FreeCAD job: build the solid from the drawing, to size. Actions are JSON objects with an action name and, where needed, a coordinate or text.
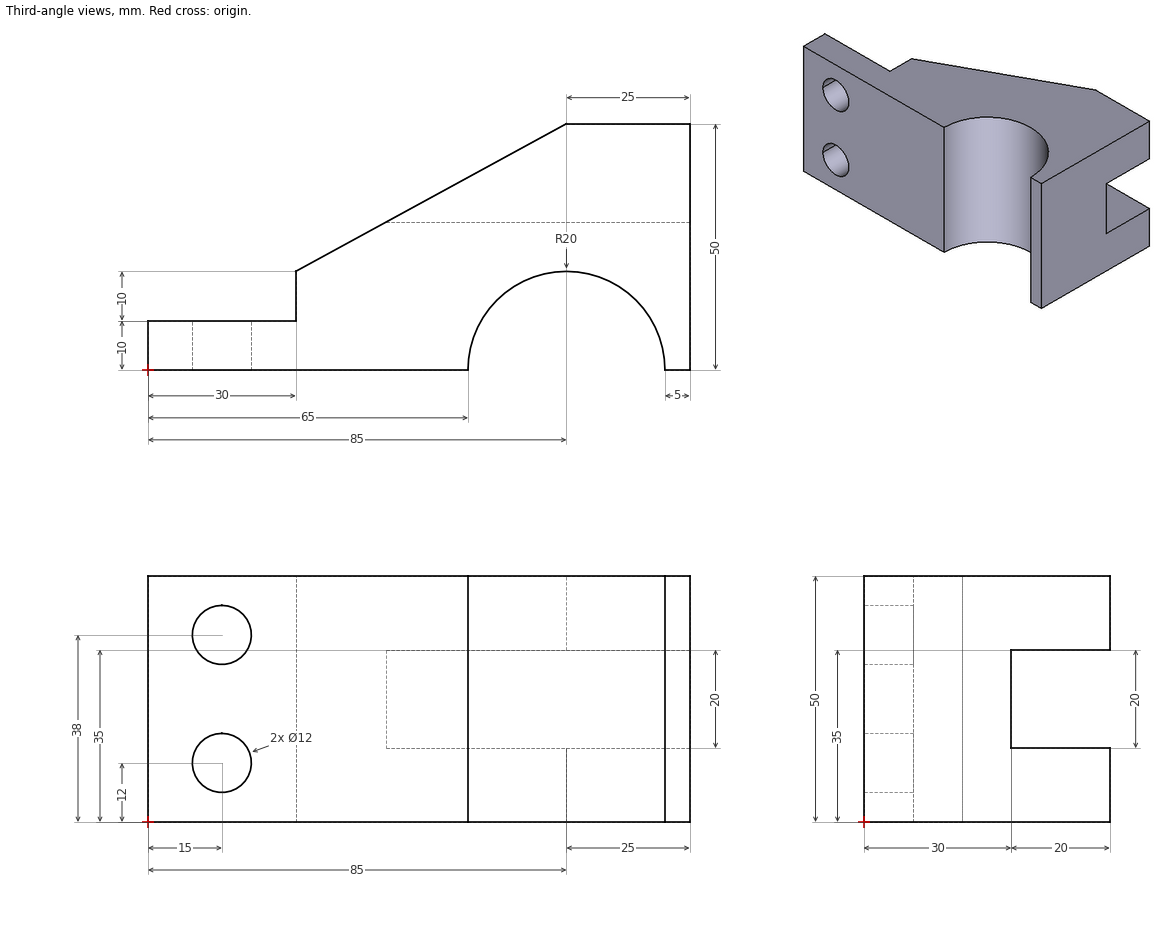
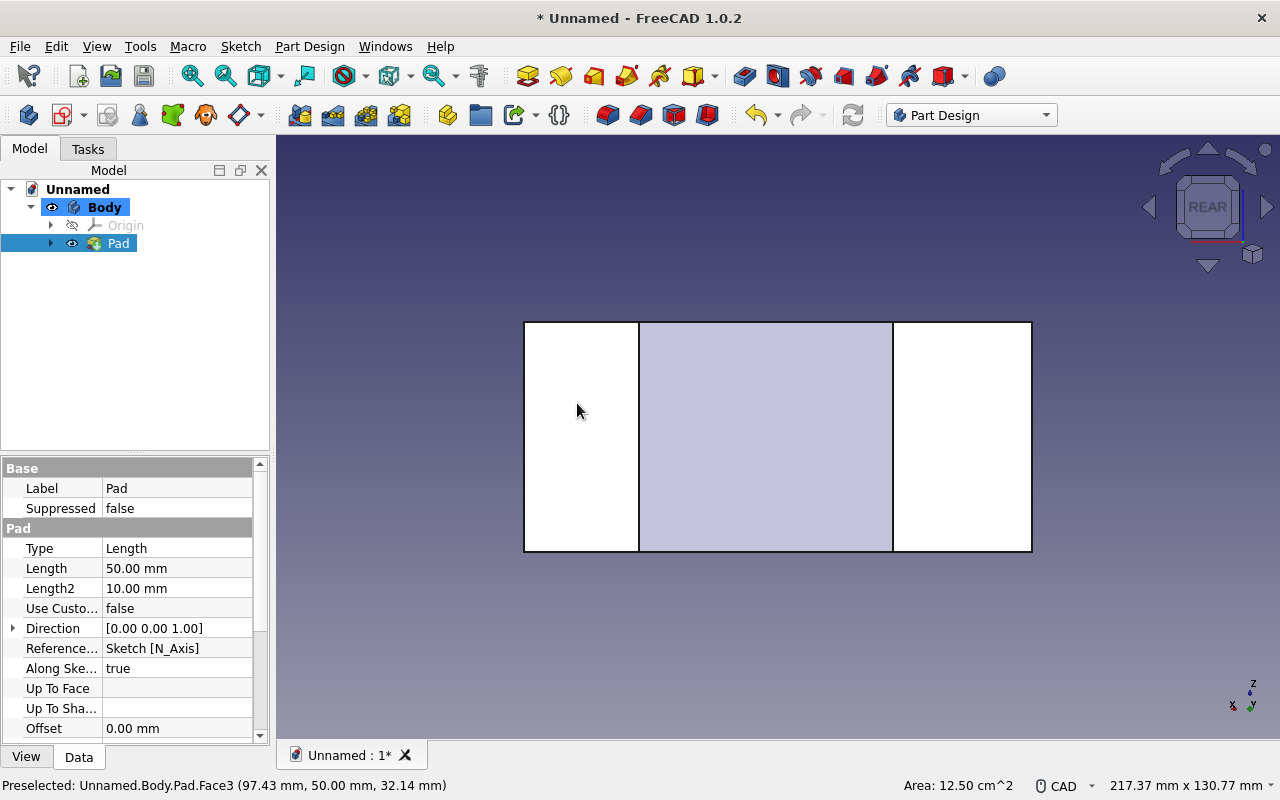
{"action": "left_click", "coordinate": [62, 116]}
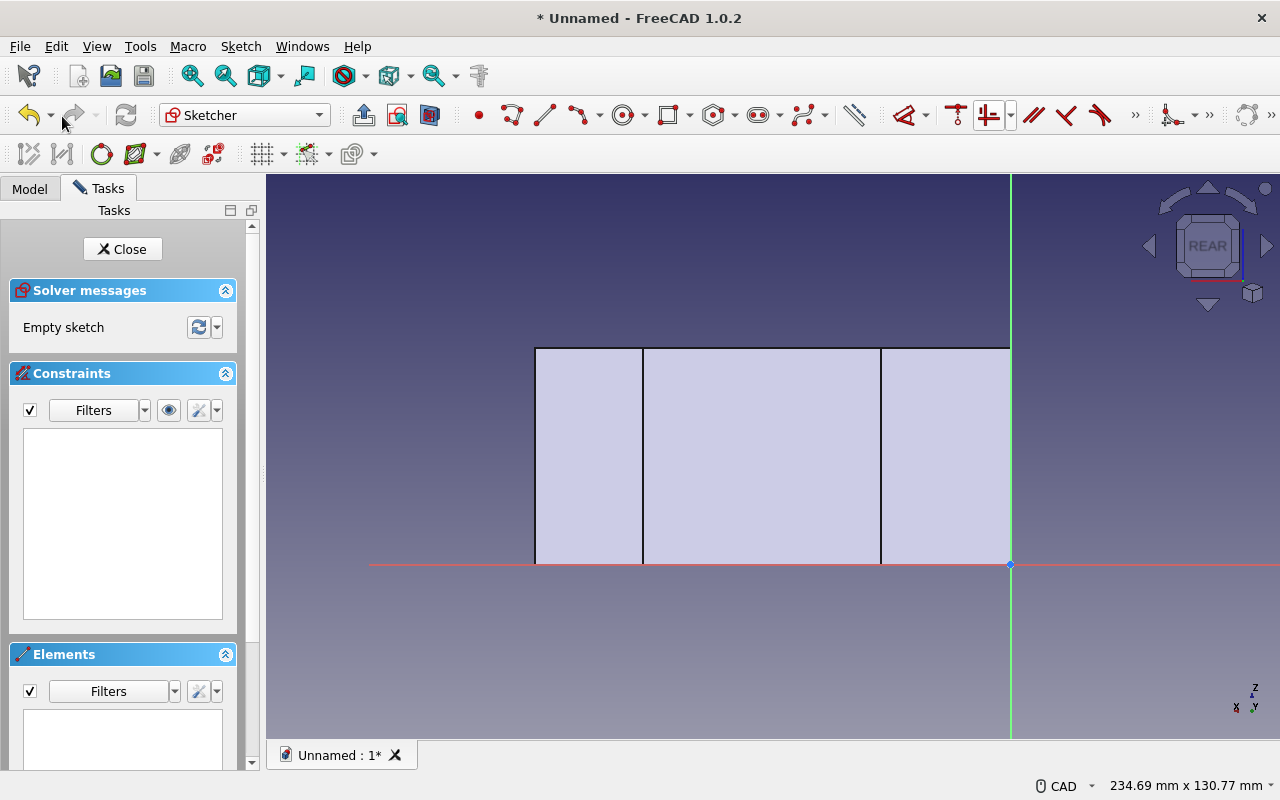
{"action": "scroll", "coordinate": [552, 456], "scroll_direction": "up", "scroll_amount": 7}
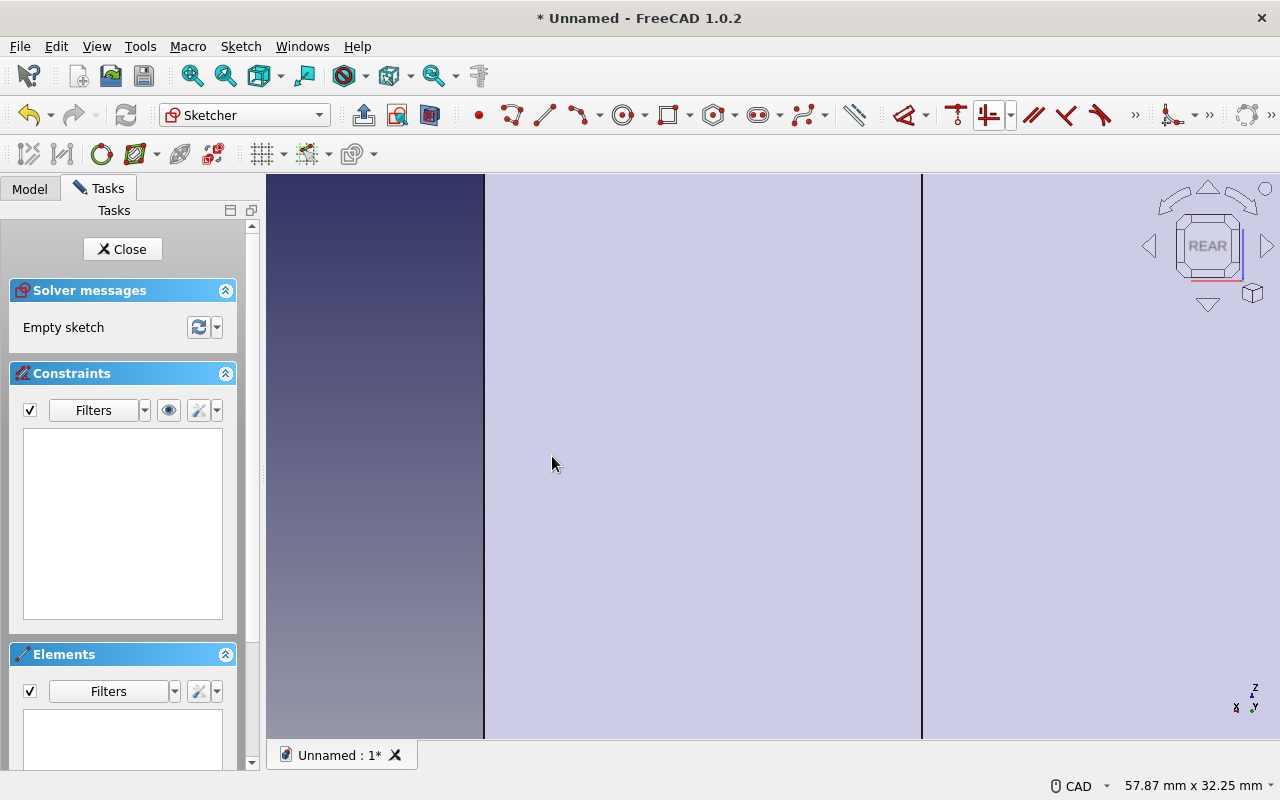
{"action": "left_click", "coordinate": [668, 116]}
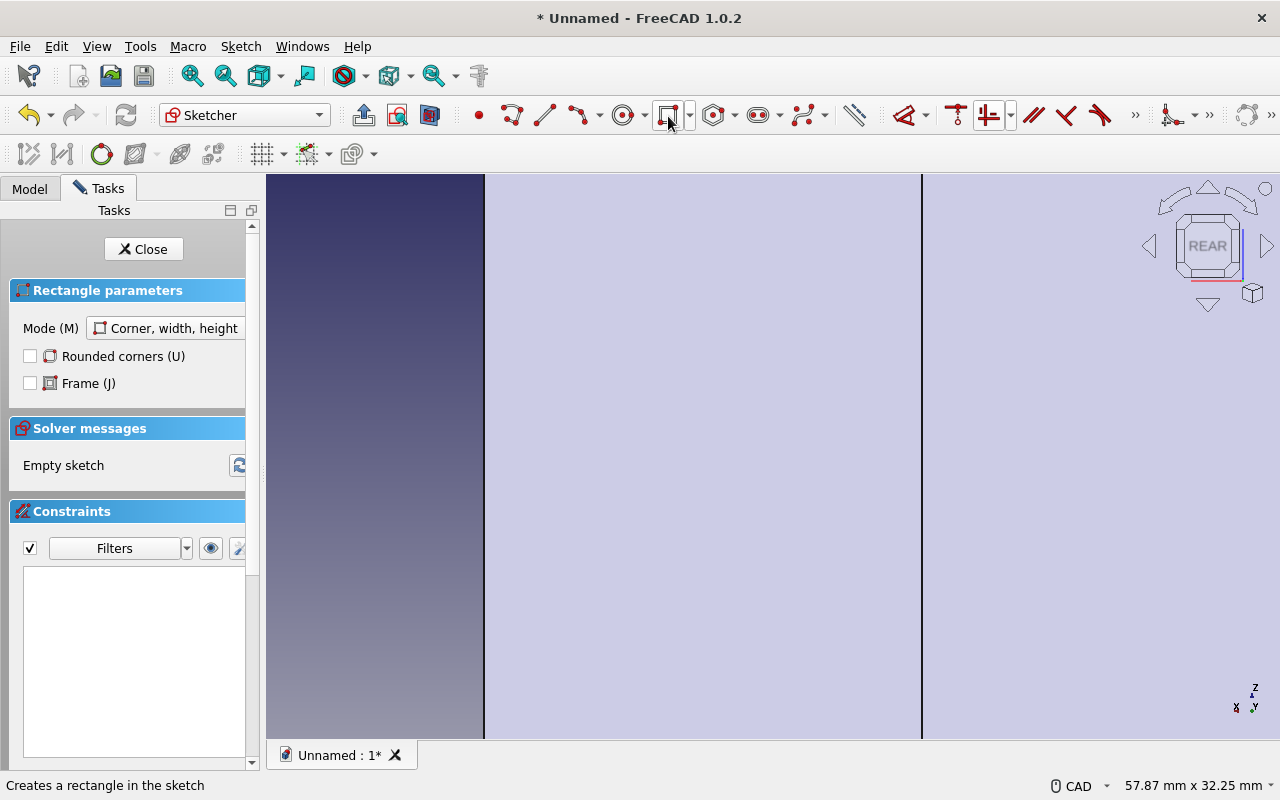
{"action": "left_click", "coordinate": [484, 281]}
{"action": "left_click", "coordinate": [922, 632]}
{"action": "key", "text": "Escape"}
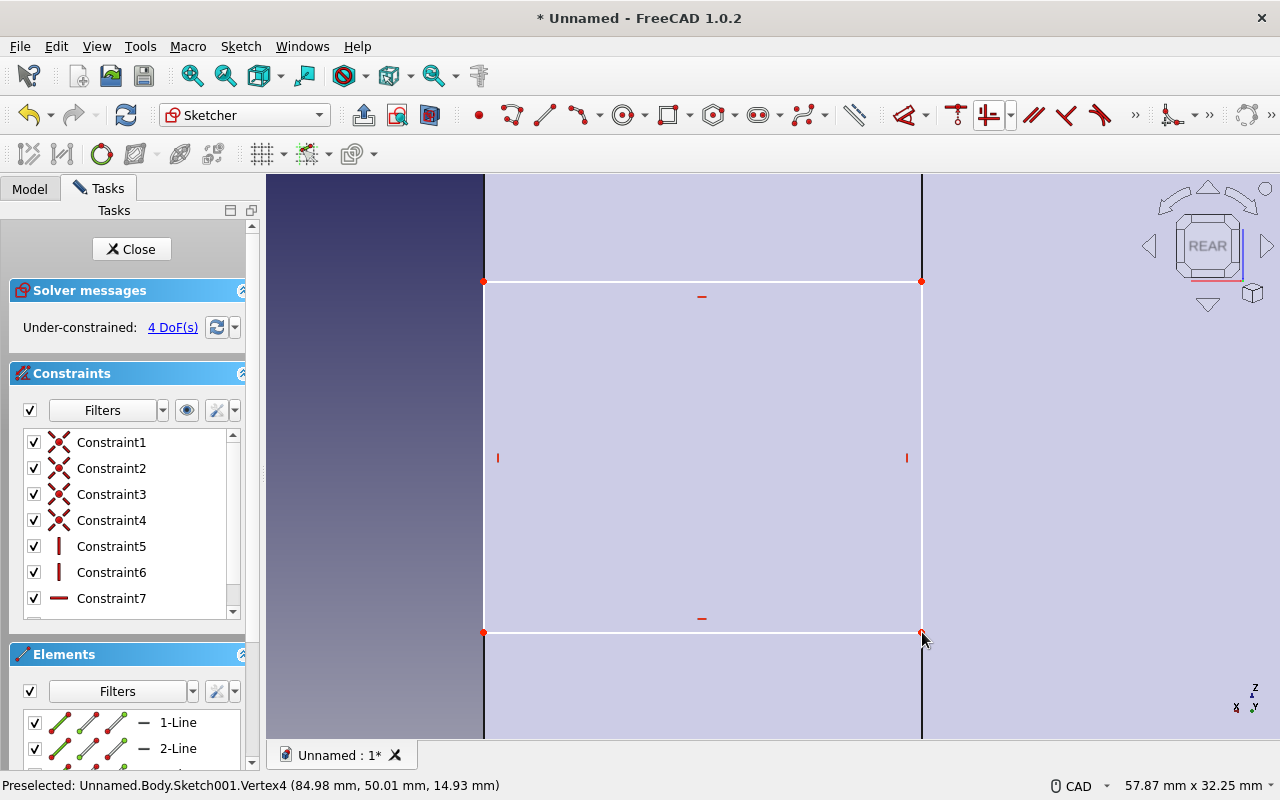
{"action": "left_click", "coordinate": [904, 116]}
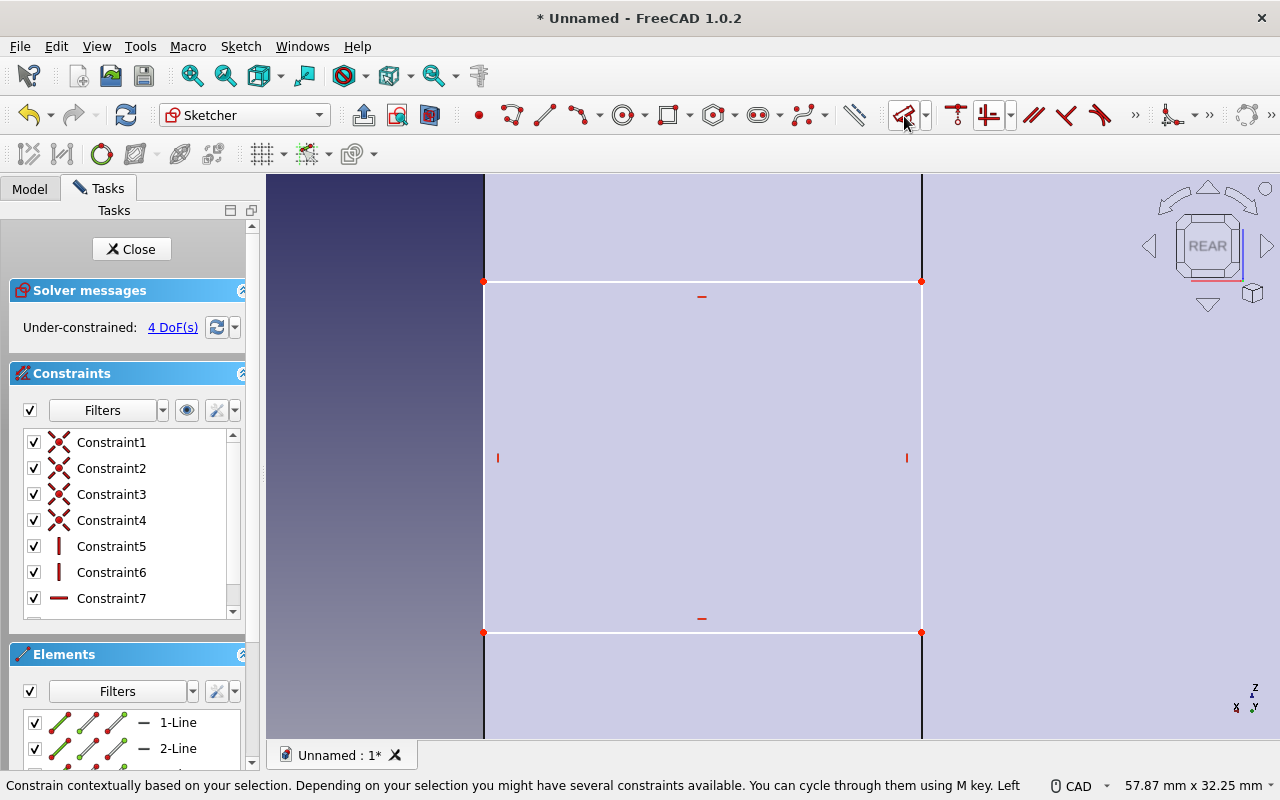
{"action": "left_click", "coordinate": [484, 387]}
{"action": "left_click", "coordinate": [450, 457]}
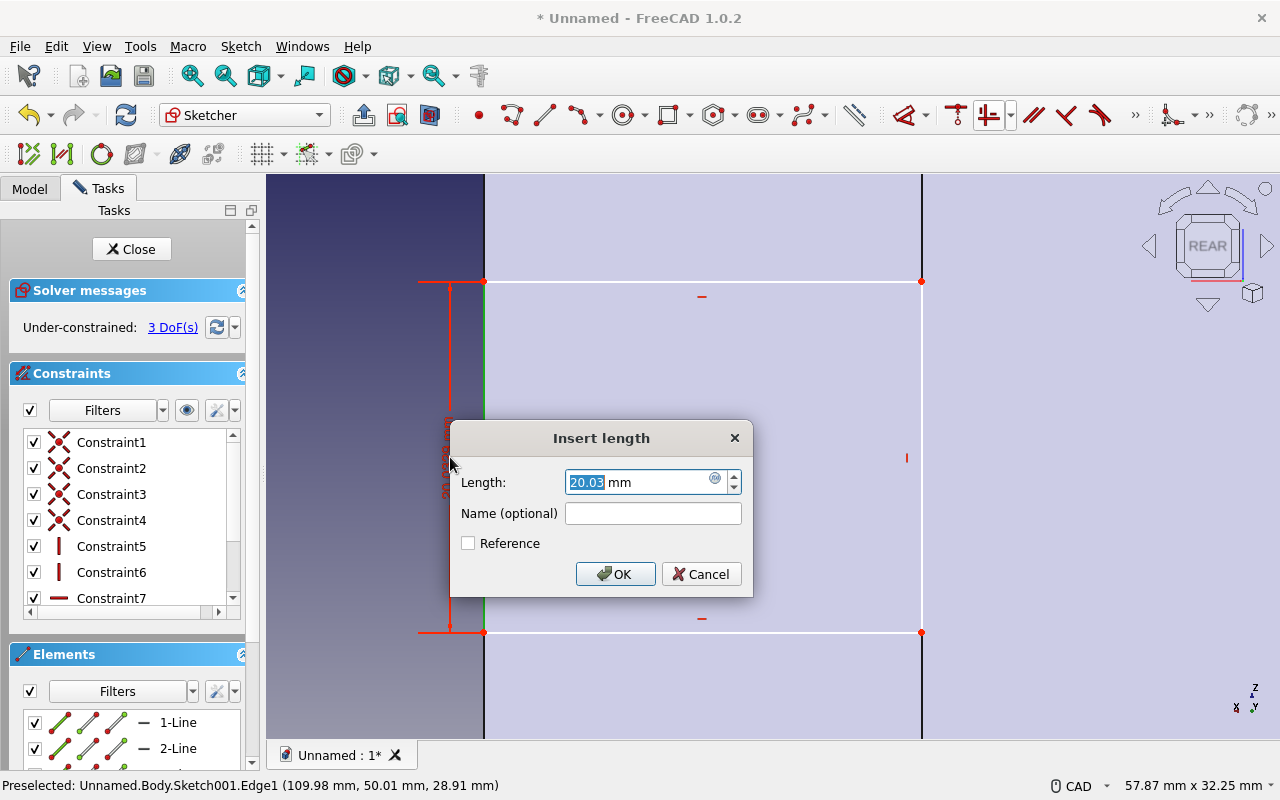
{"action": "type", "text": "20"}
{"action": "key", "text": "Return"}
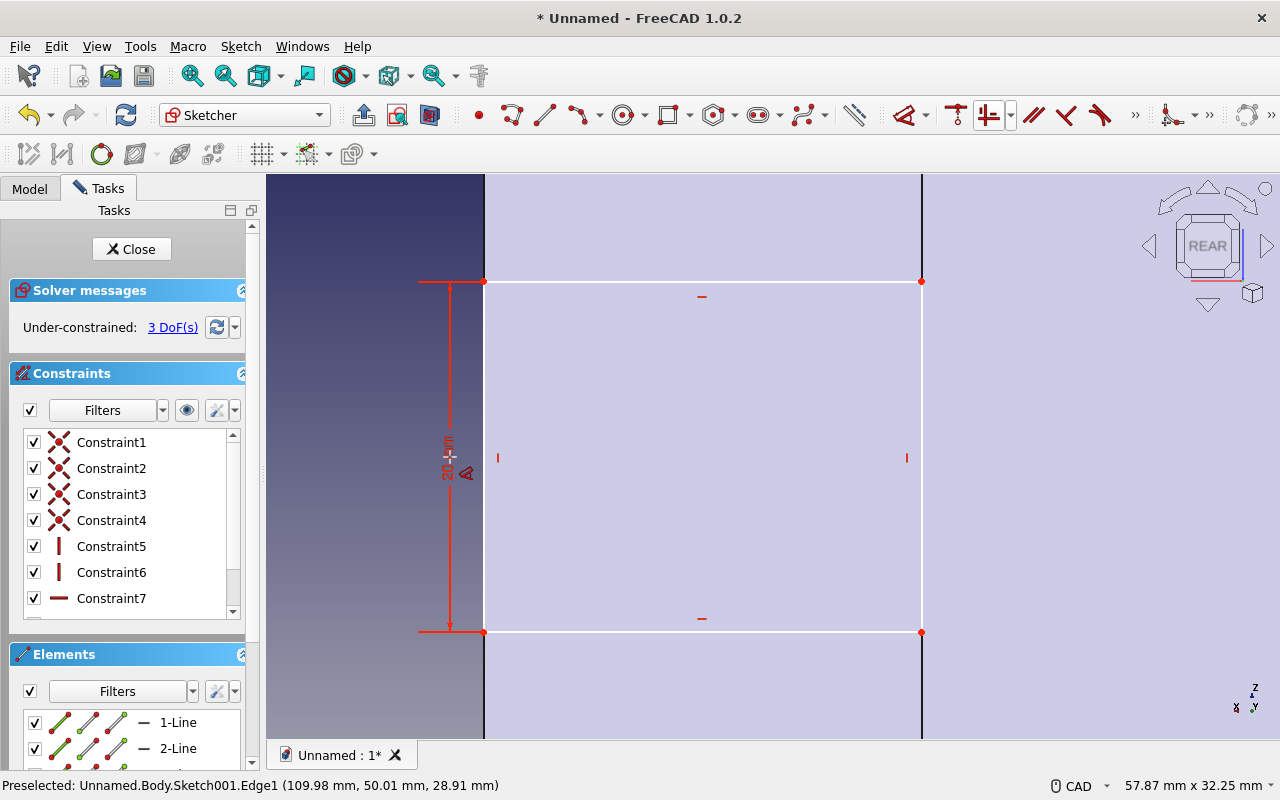
{"action": "left_click", "coordinate": [615, 632]}
{"action": "left_click", "coordinate": [703, 666]}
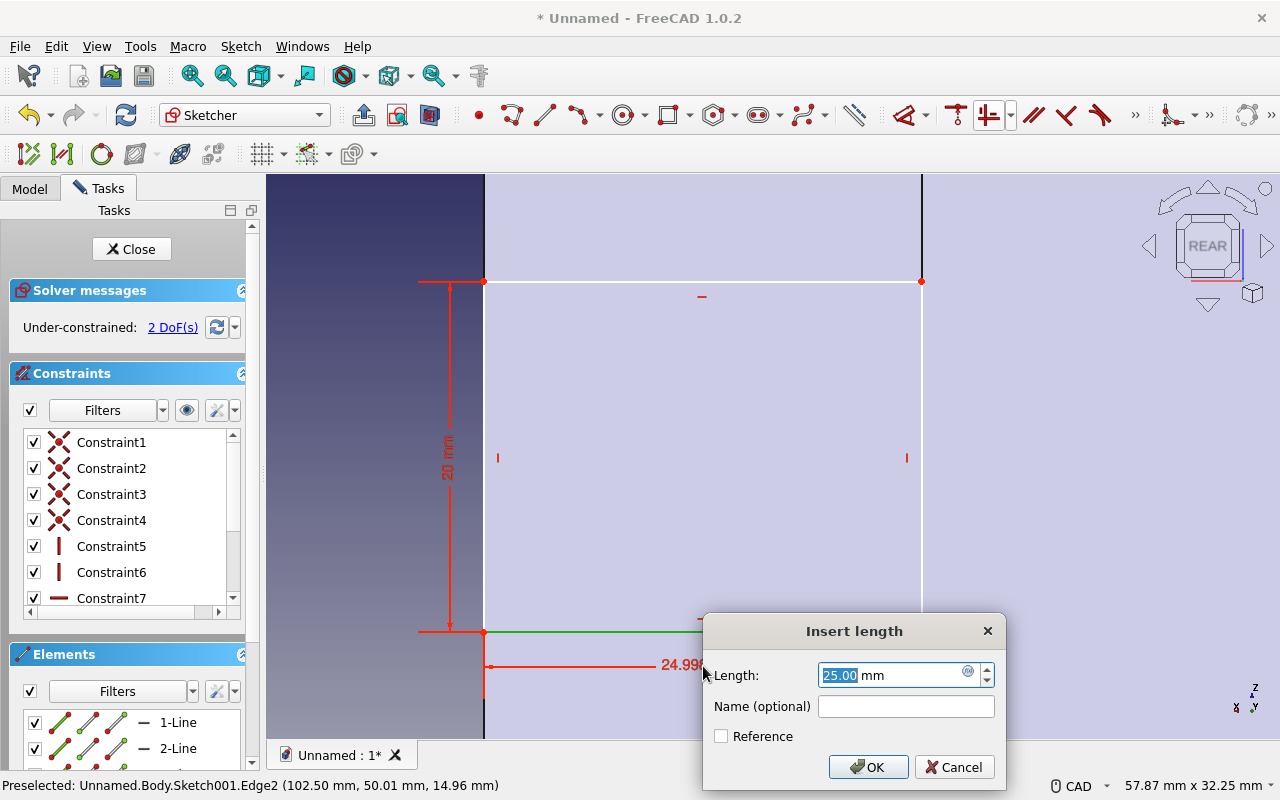
{"action": "type", "text": "25"}
{"action": "key", "text": "Return"}